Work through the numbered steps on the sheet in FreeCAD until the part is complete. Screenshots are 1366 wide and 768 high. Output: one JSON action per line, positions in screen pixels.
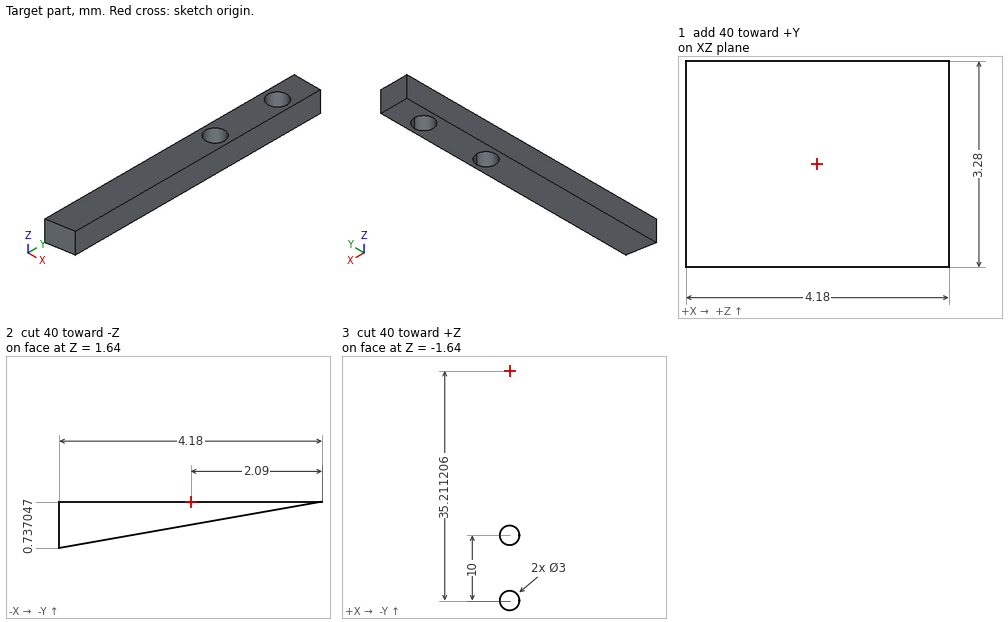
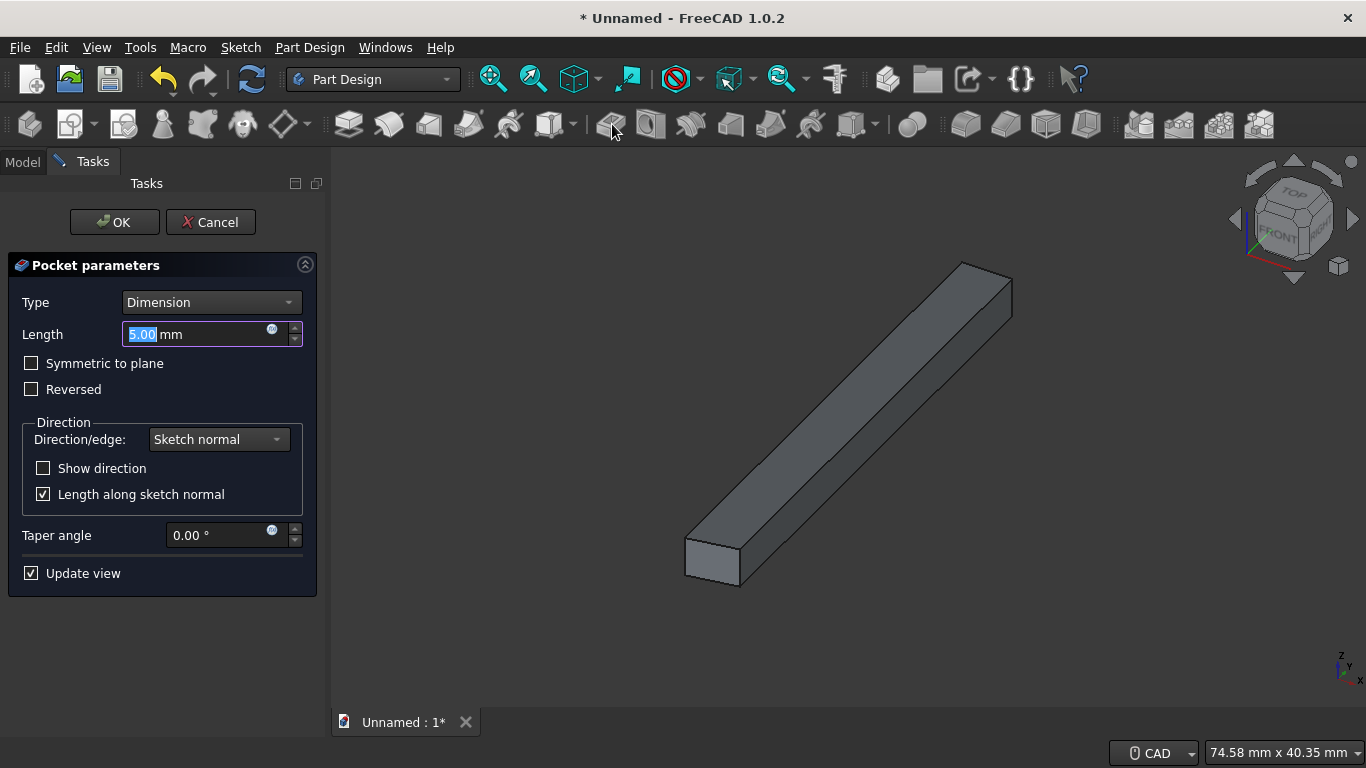
{"action": "type", "text": "40"}
{"action": "key", "text": "Tab"}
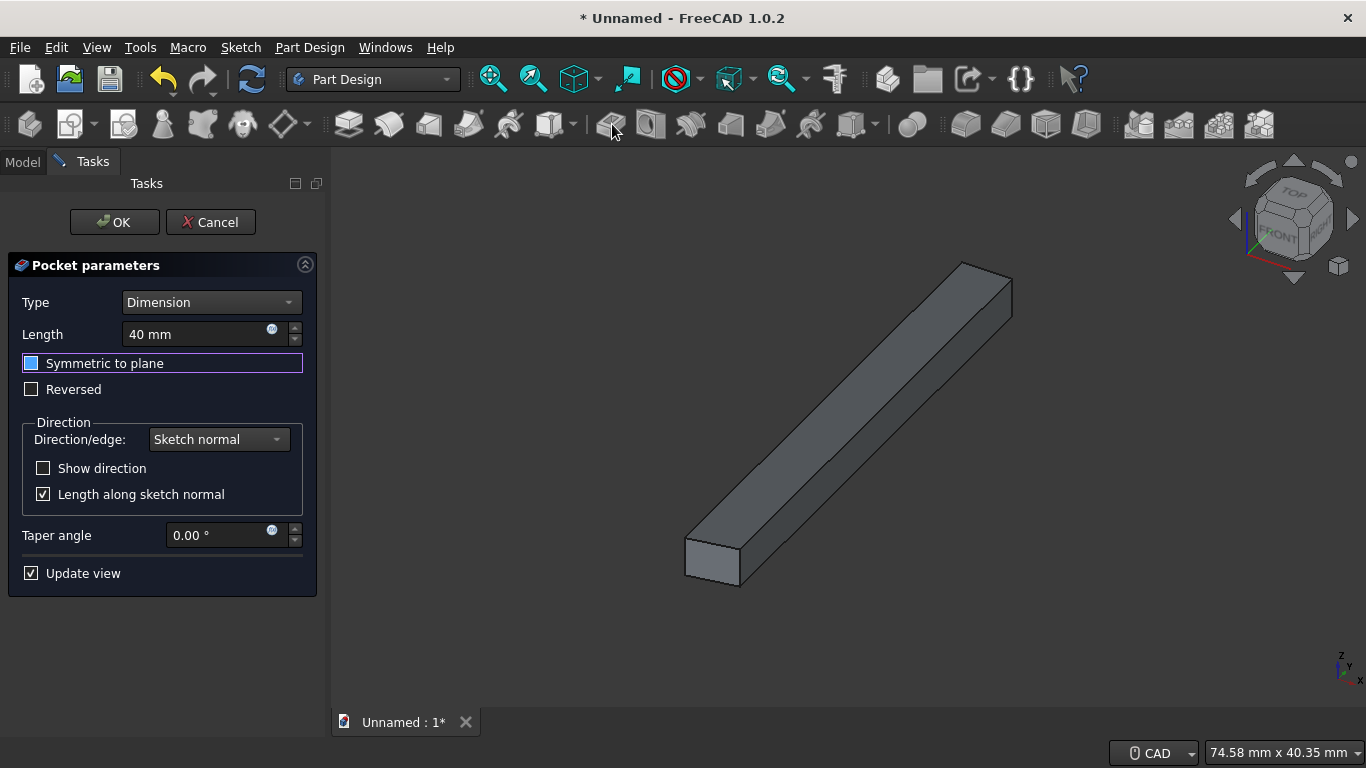
{"action": "left_click", "coordinate": [115, 222]}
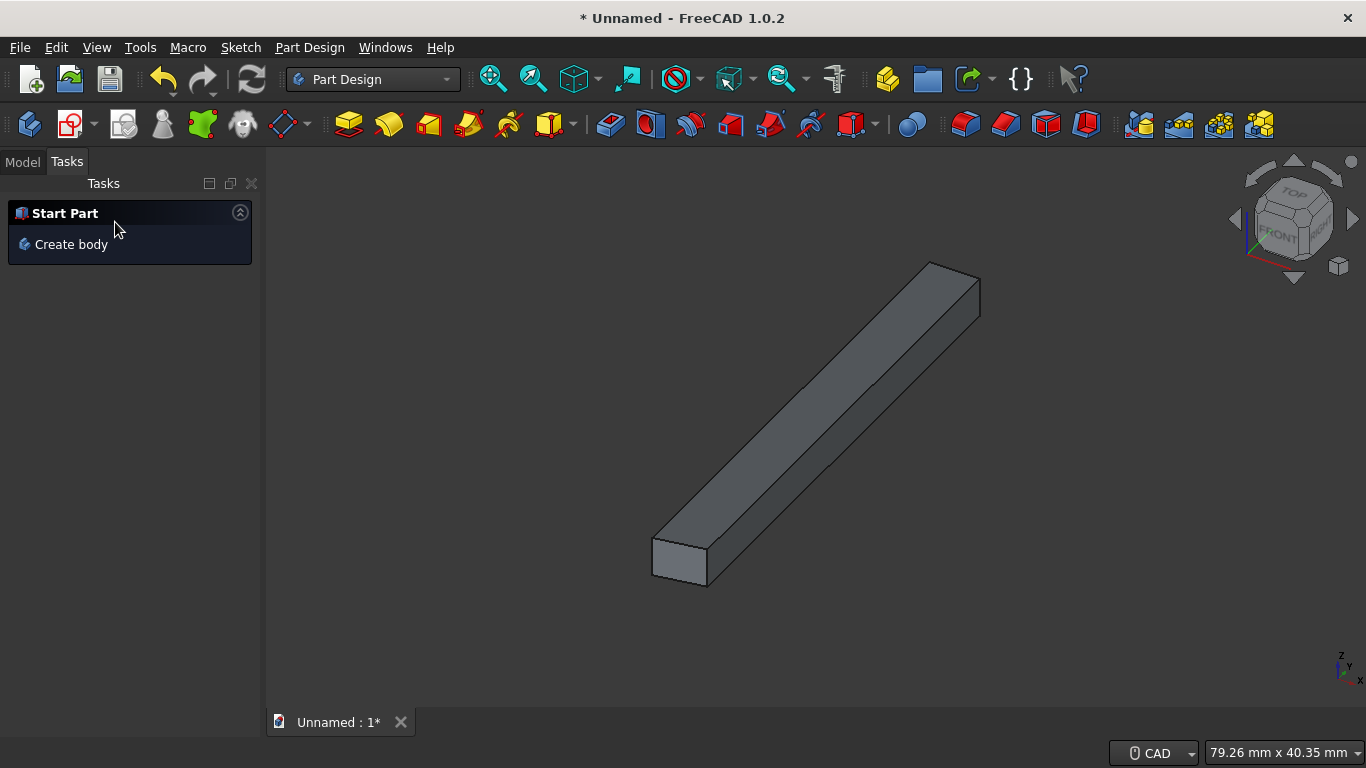
{"action": "key", "text": "5"}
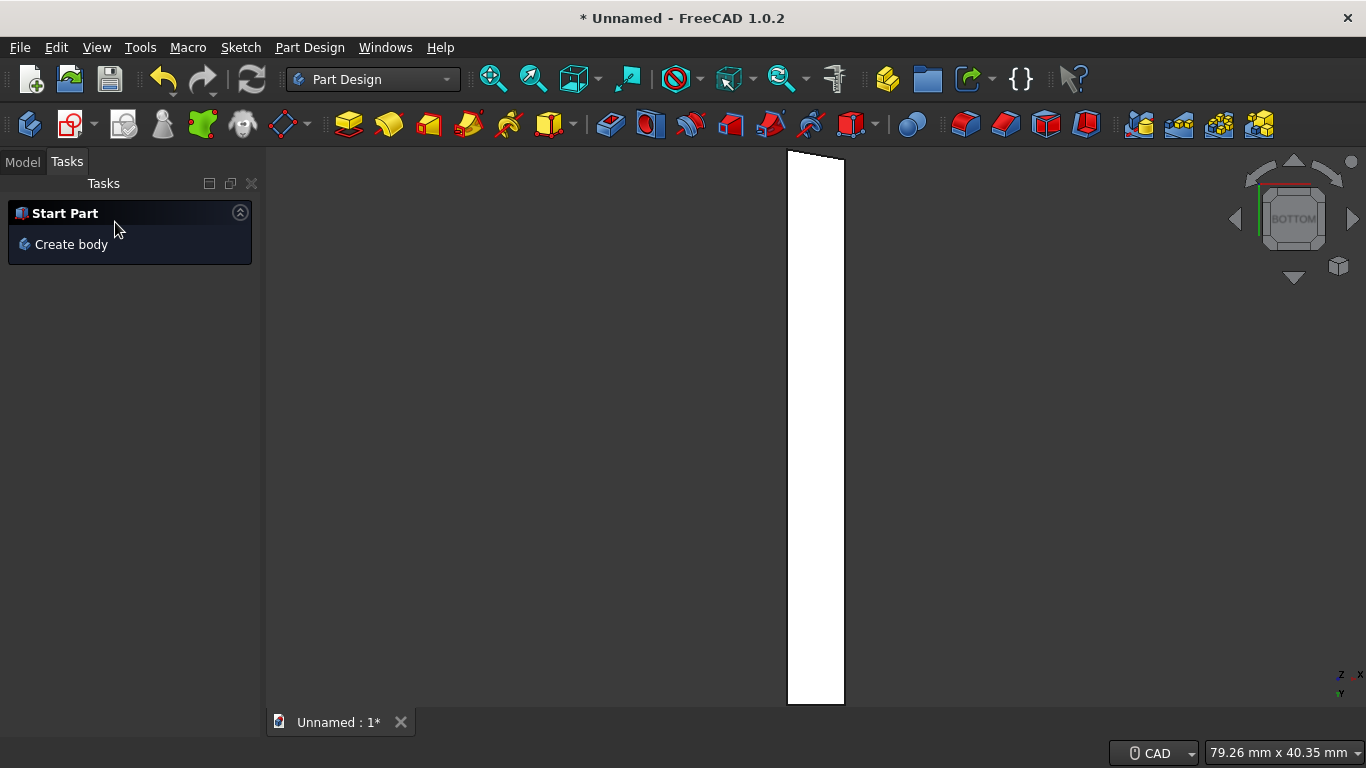
{"action": "left_click", "coordinate": [816, 664]}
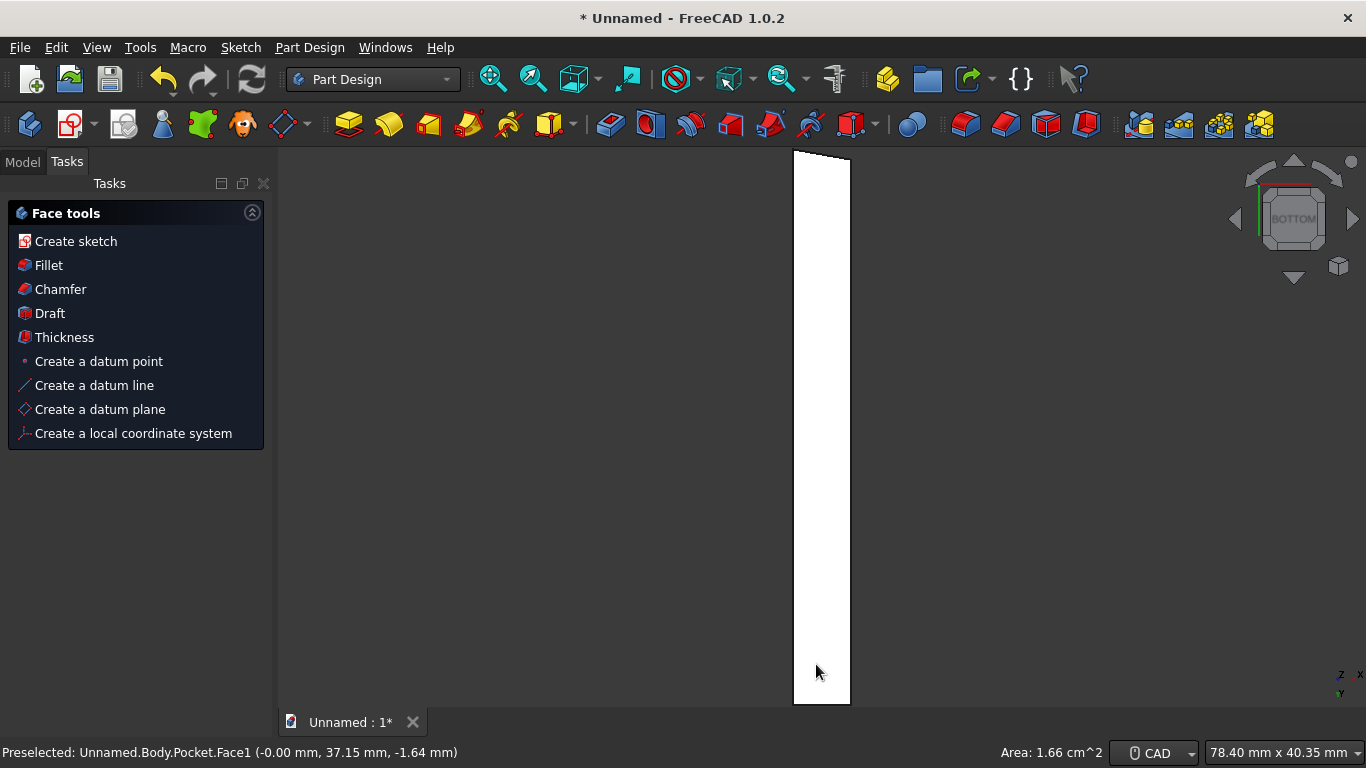
{"action": "left_click", "coordinate": [70, 124]}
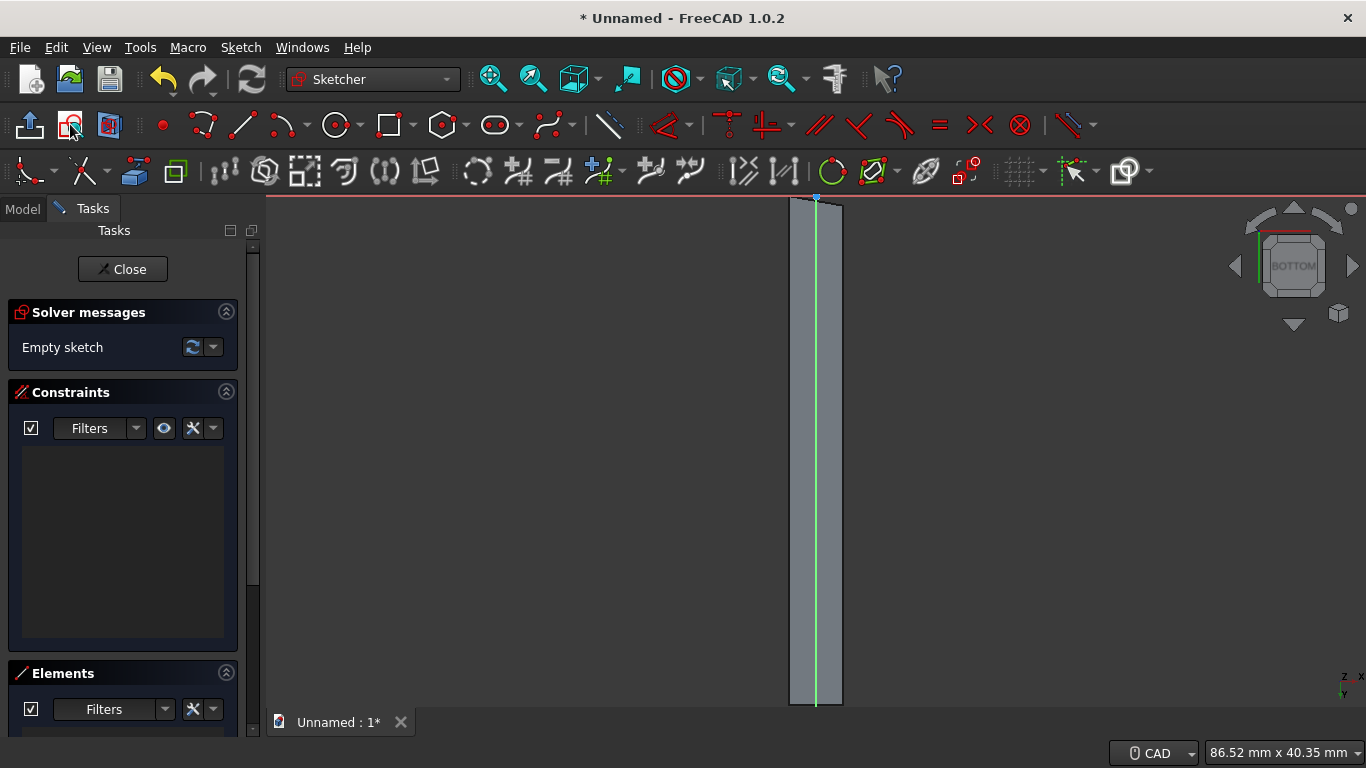
{"action": "scroll", "coordinate": [899, 679], "scroll_direction": "up", "scroll_amount": 3}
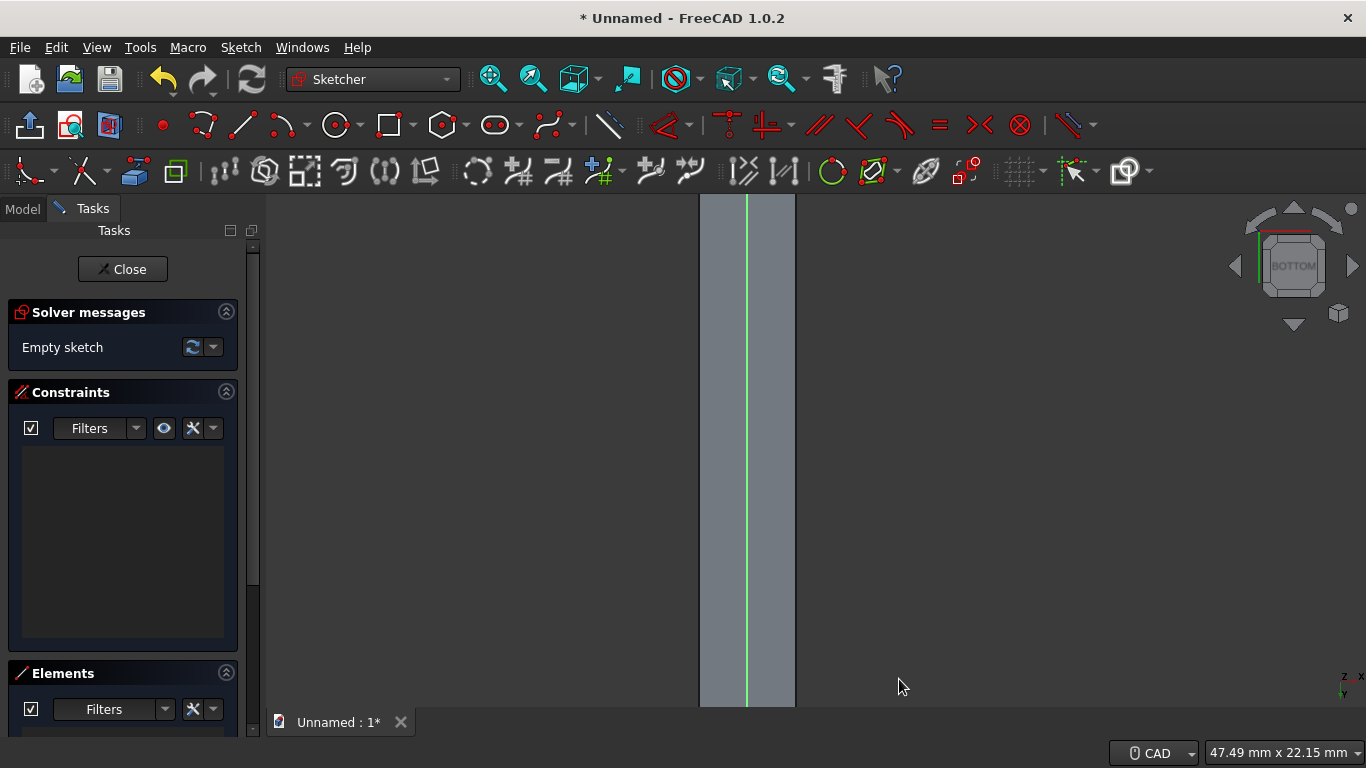
{"action": "left_click", "coordinate": [336, 126]}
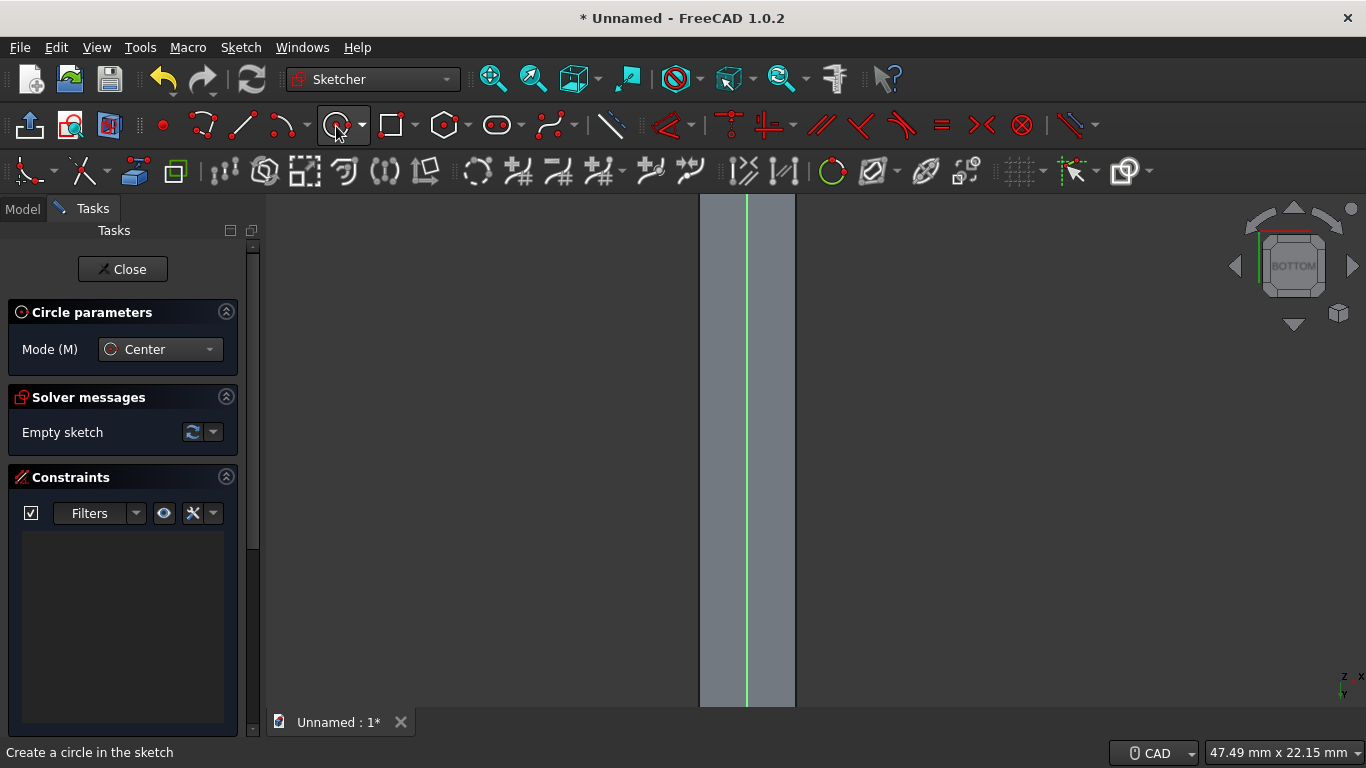
{"action": "left_click", "coordinate": [747, 614]}
{"action": "mouse_move", "coordinate": [772, 590]}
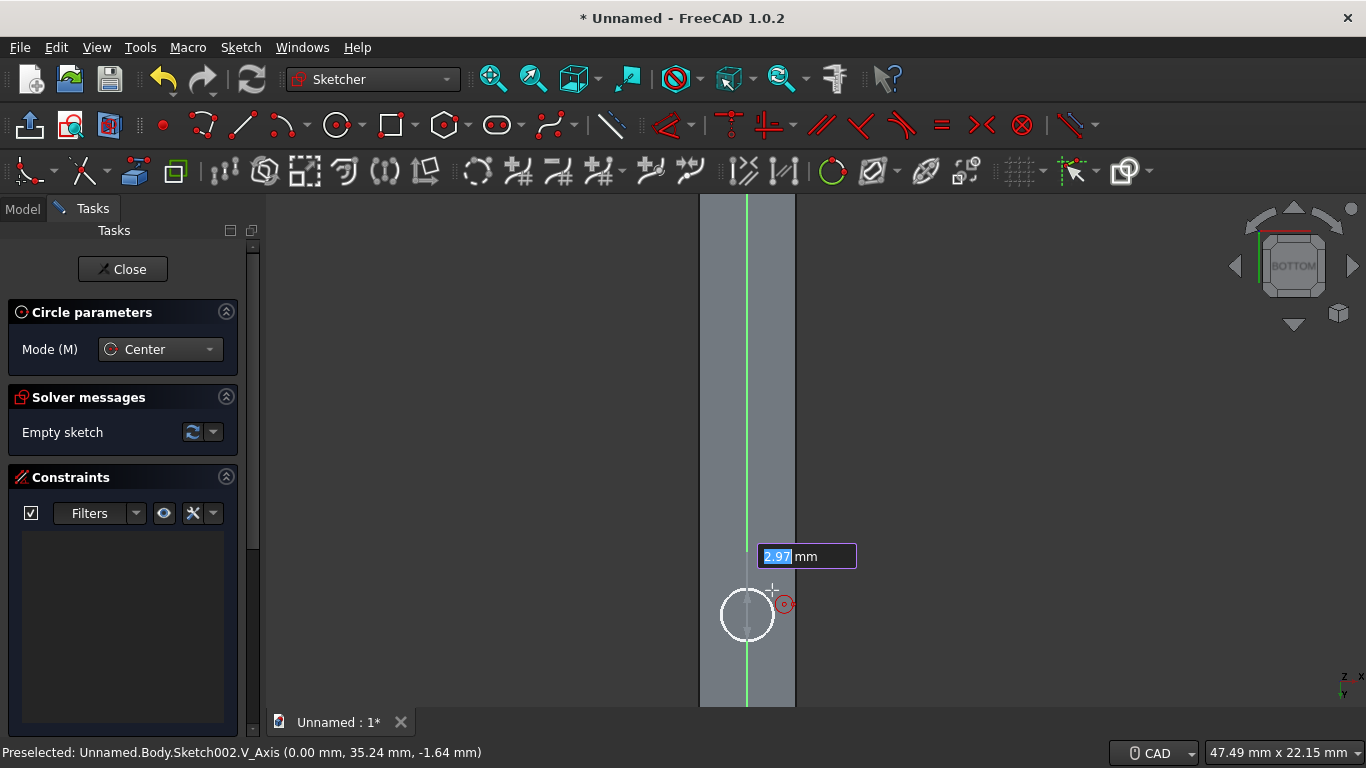
{"action": "type", "text": "3"}
{"action": "key", "text": "Return"}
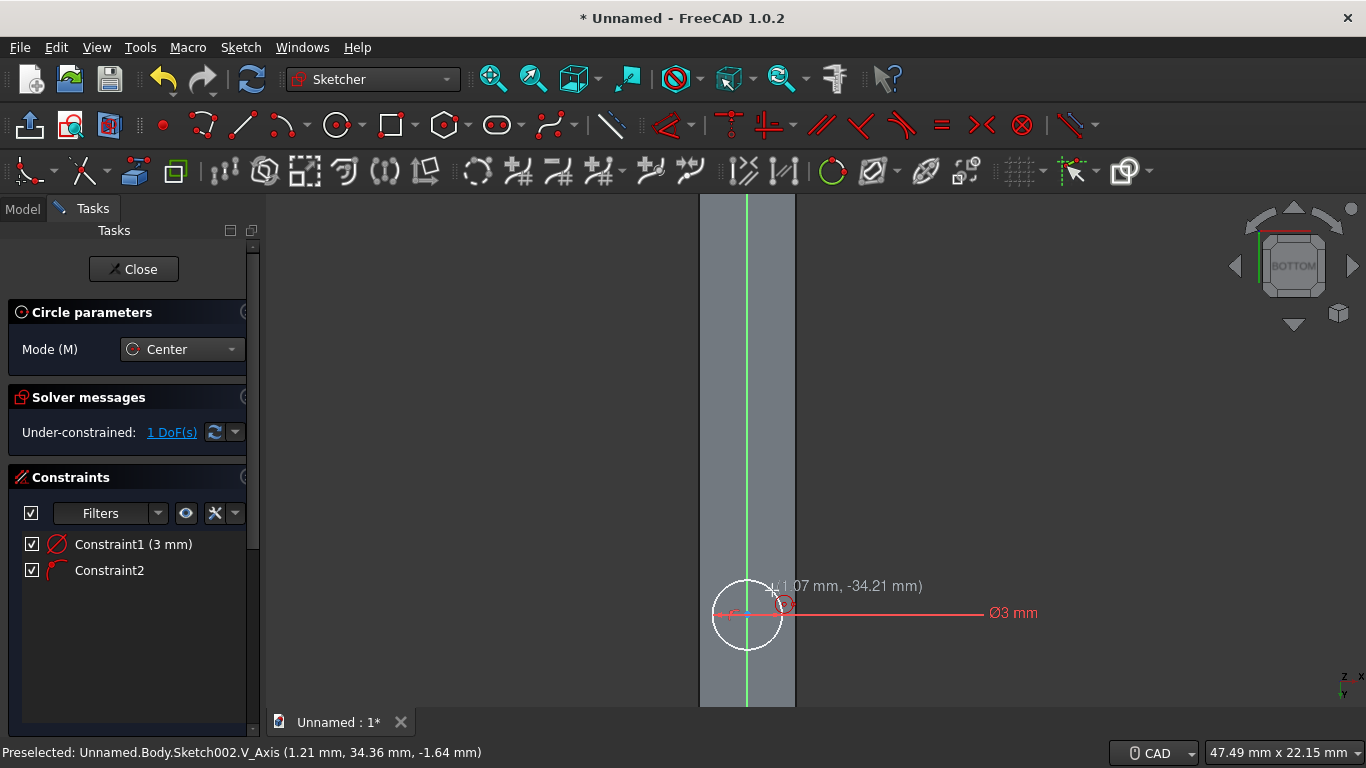
{"action": "left_click", "coordinate": [747, 383]}
{"action": "mouse_move", "coordinate": [772, 358]}